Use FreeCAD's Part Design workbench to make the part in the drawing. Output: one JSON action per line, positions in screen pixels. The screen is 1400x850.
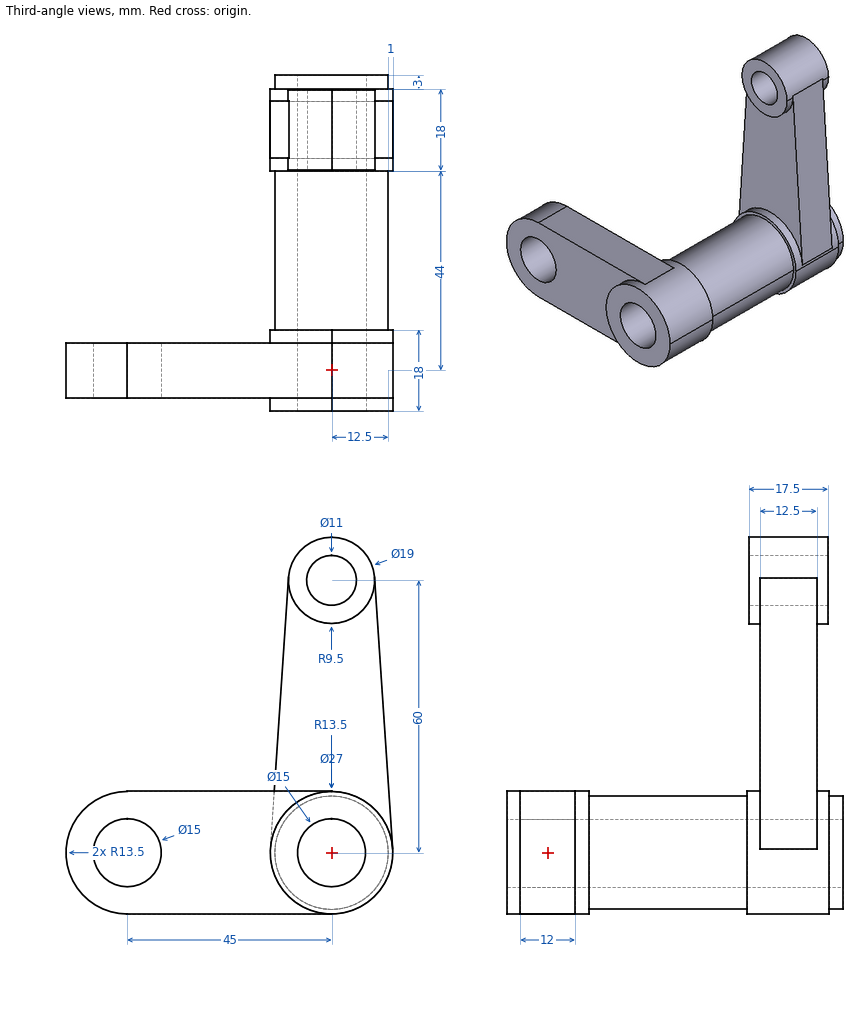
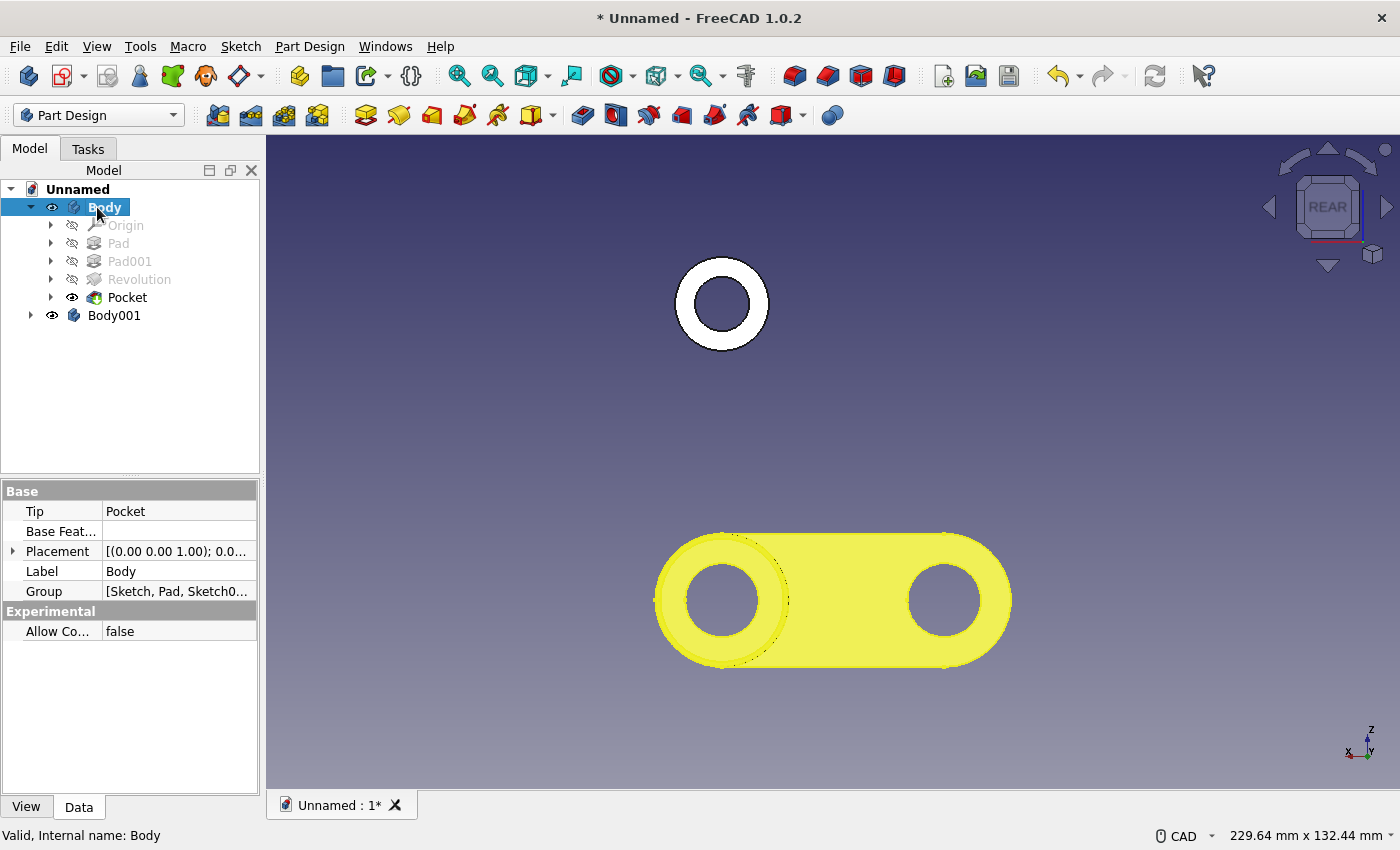
{"action": "left_click", "coordinate": [148, 631]}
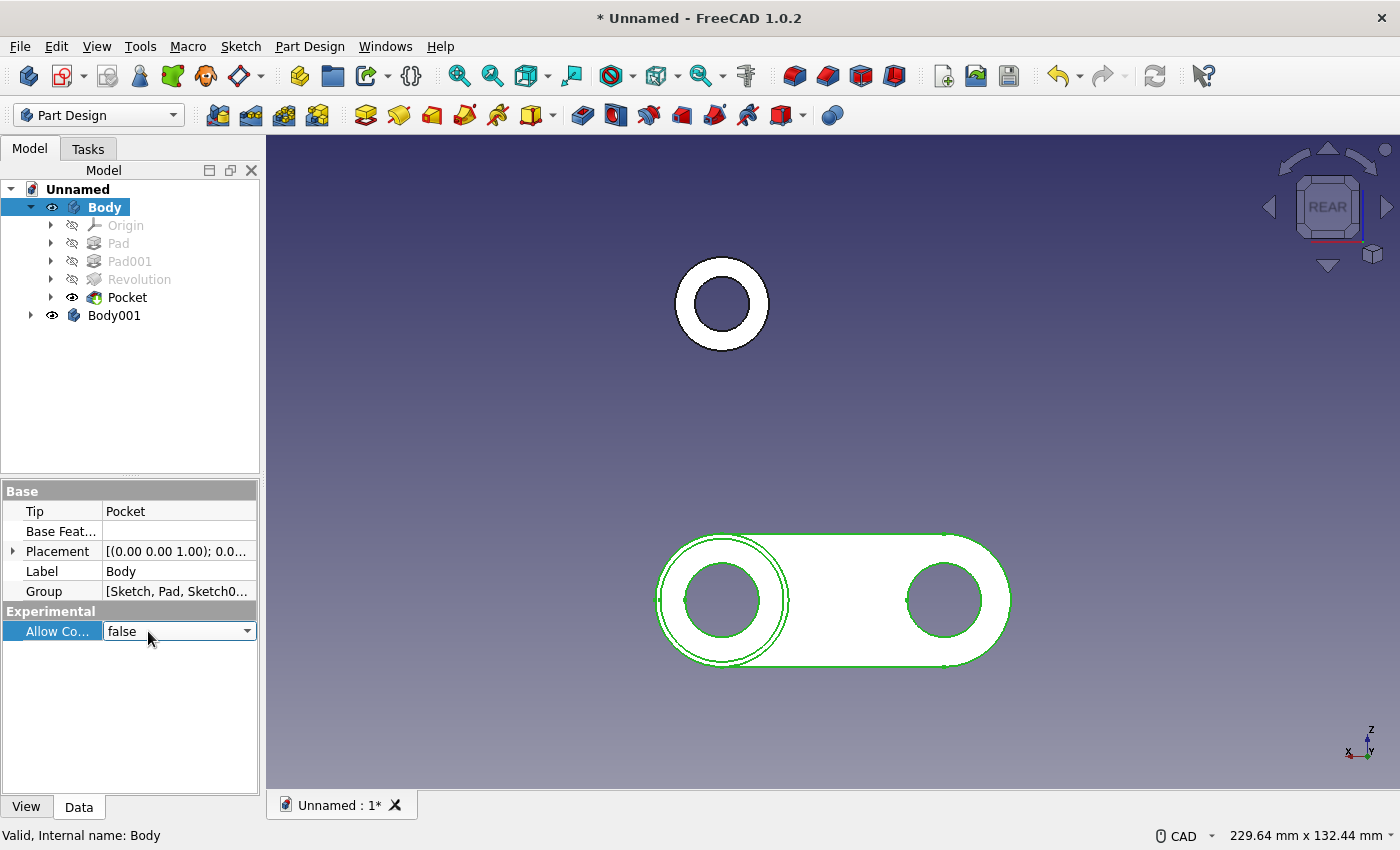
{"action": "left_click", "coordinate": [148, 631]}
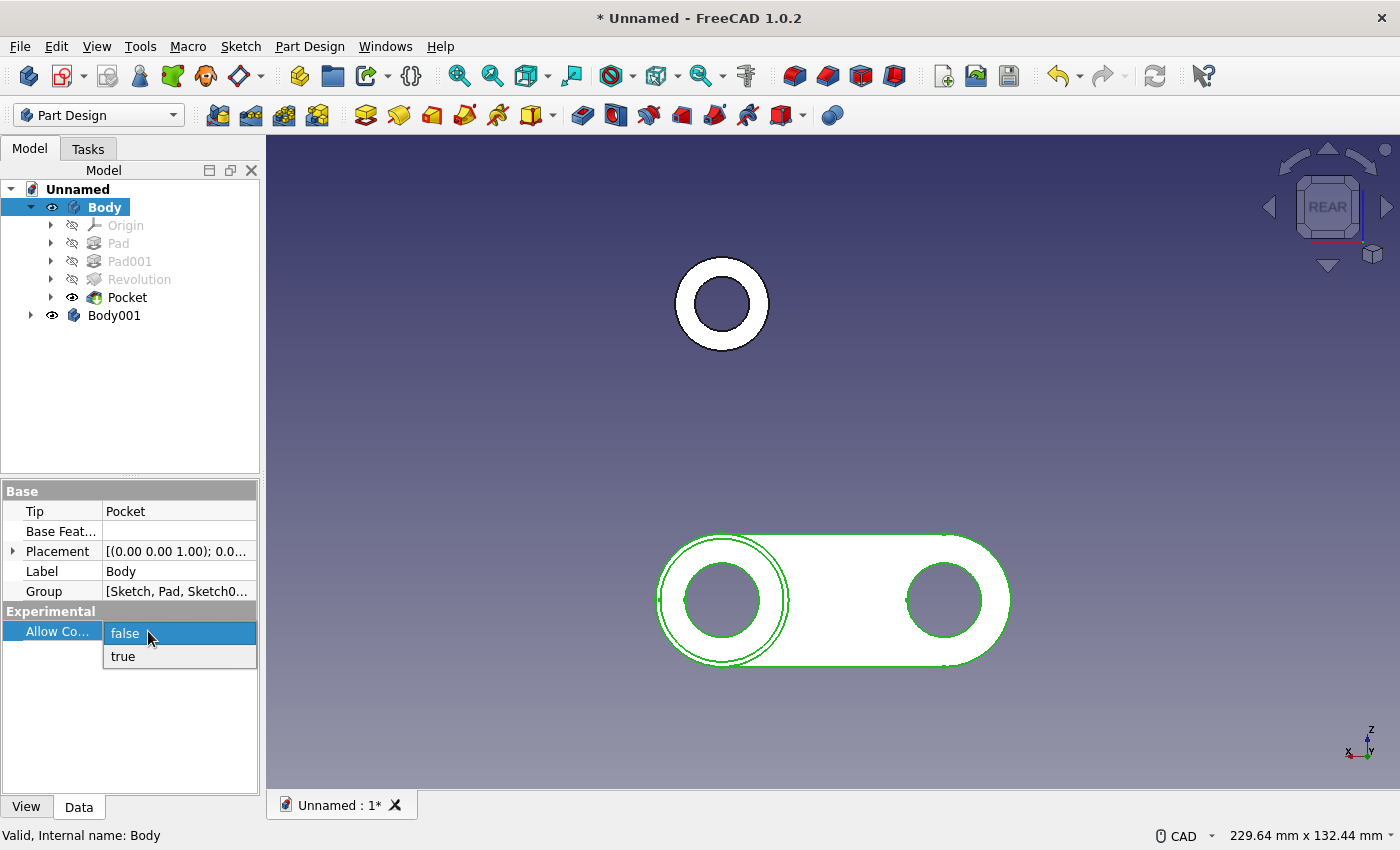
{"action": "left_click", "coordinate": [178, 656]}
{"action": "key", "text": "Return"}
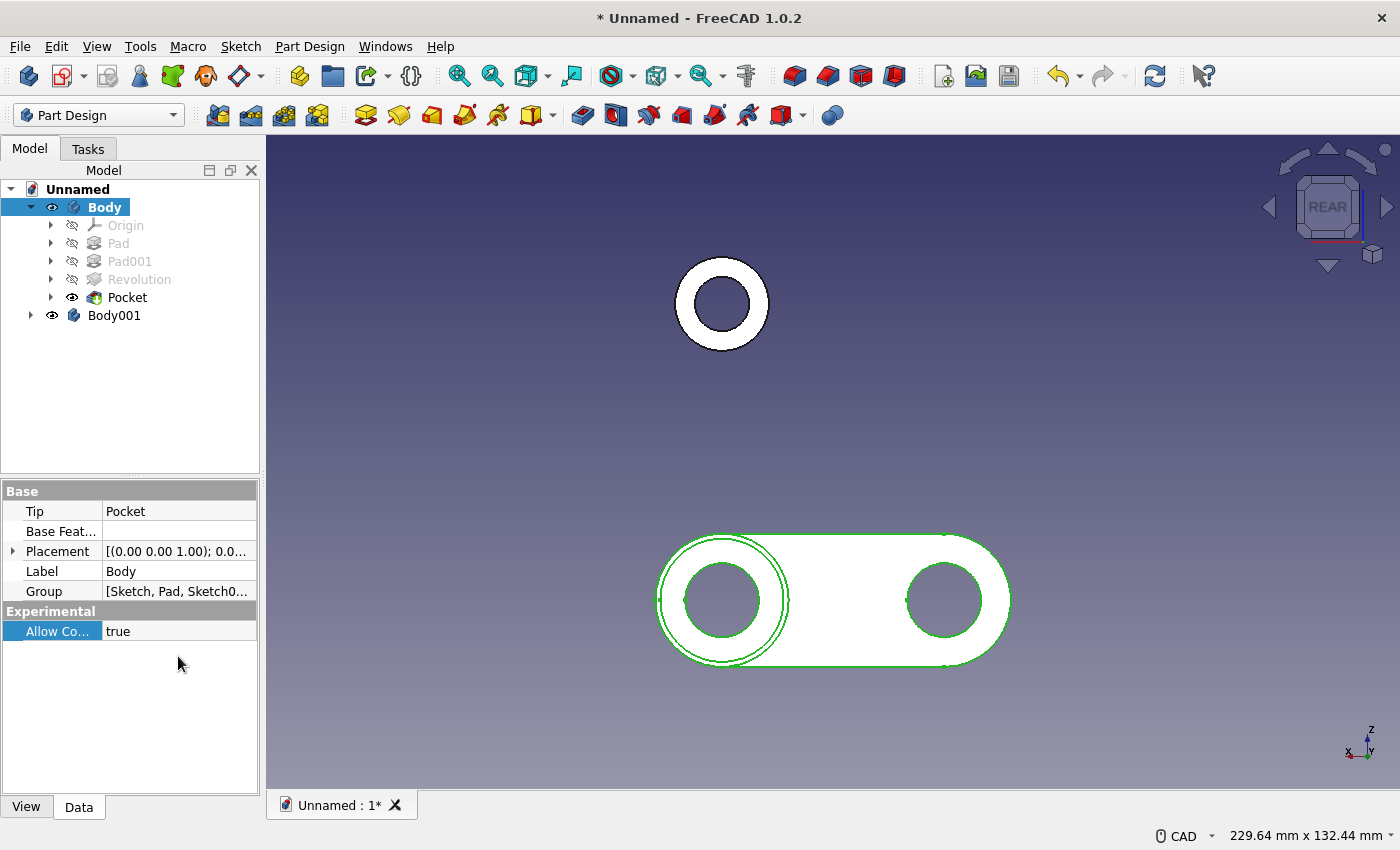
{"action": "left_click", "coordinate": [97, 315]}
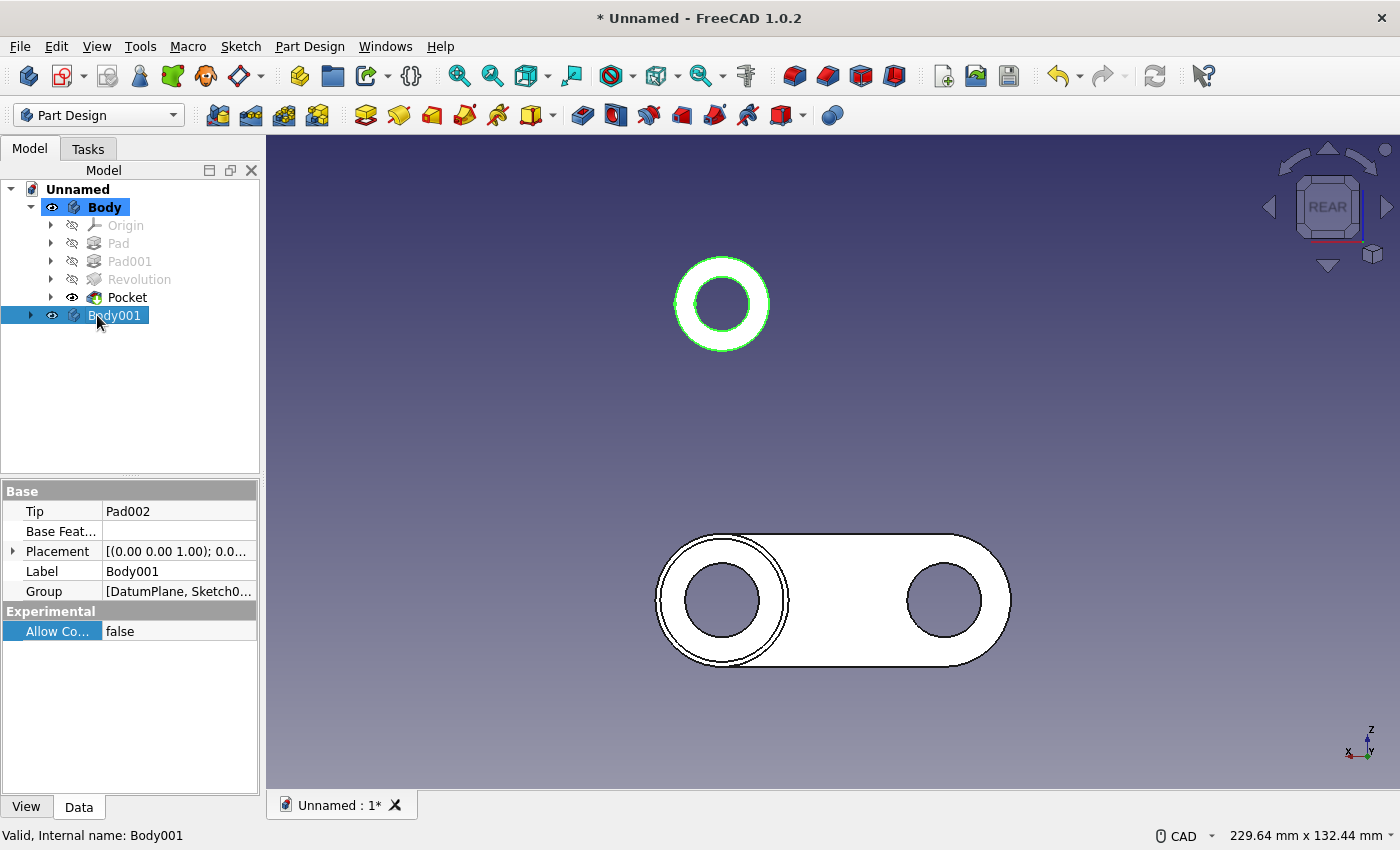
{"action": "left_click", "coordinate": [833, 116]}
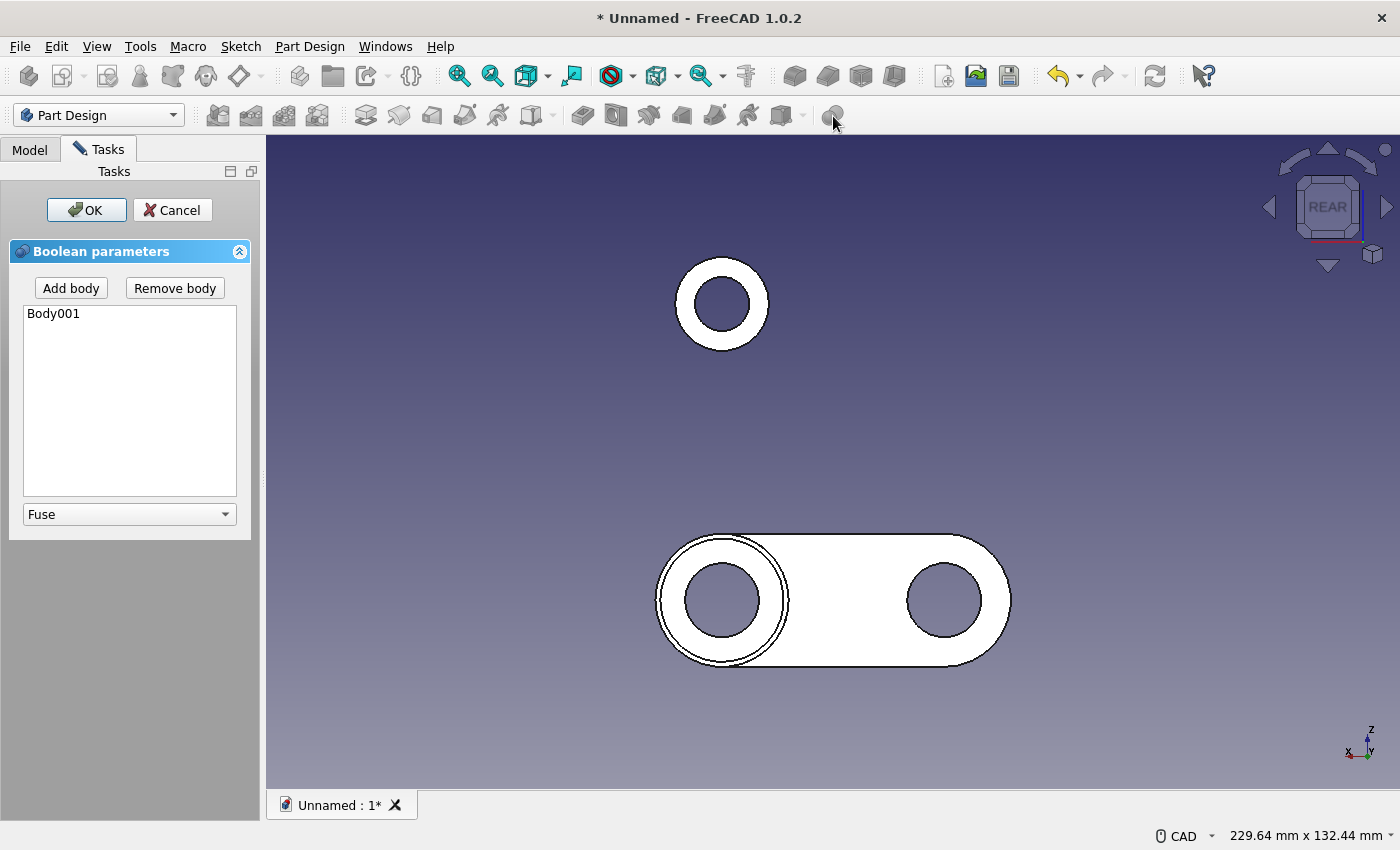
{"action": "left_click", "coordinate": [87, 210]}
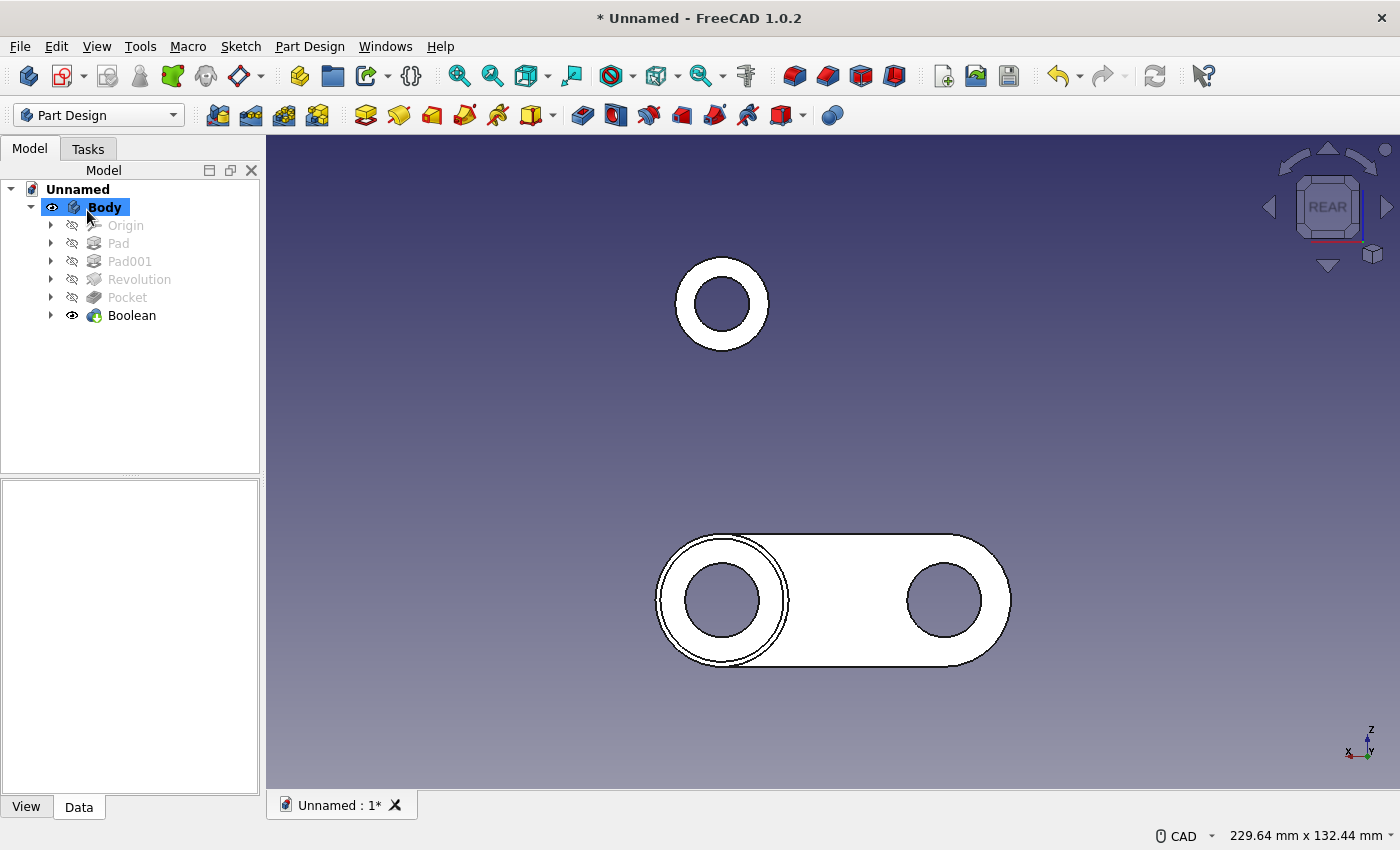
{"action": "left_click", "coordinate": [51, 225]}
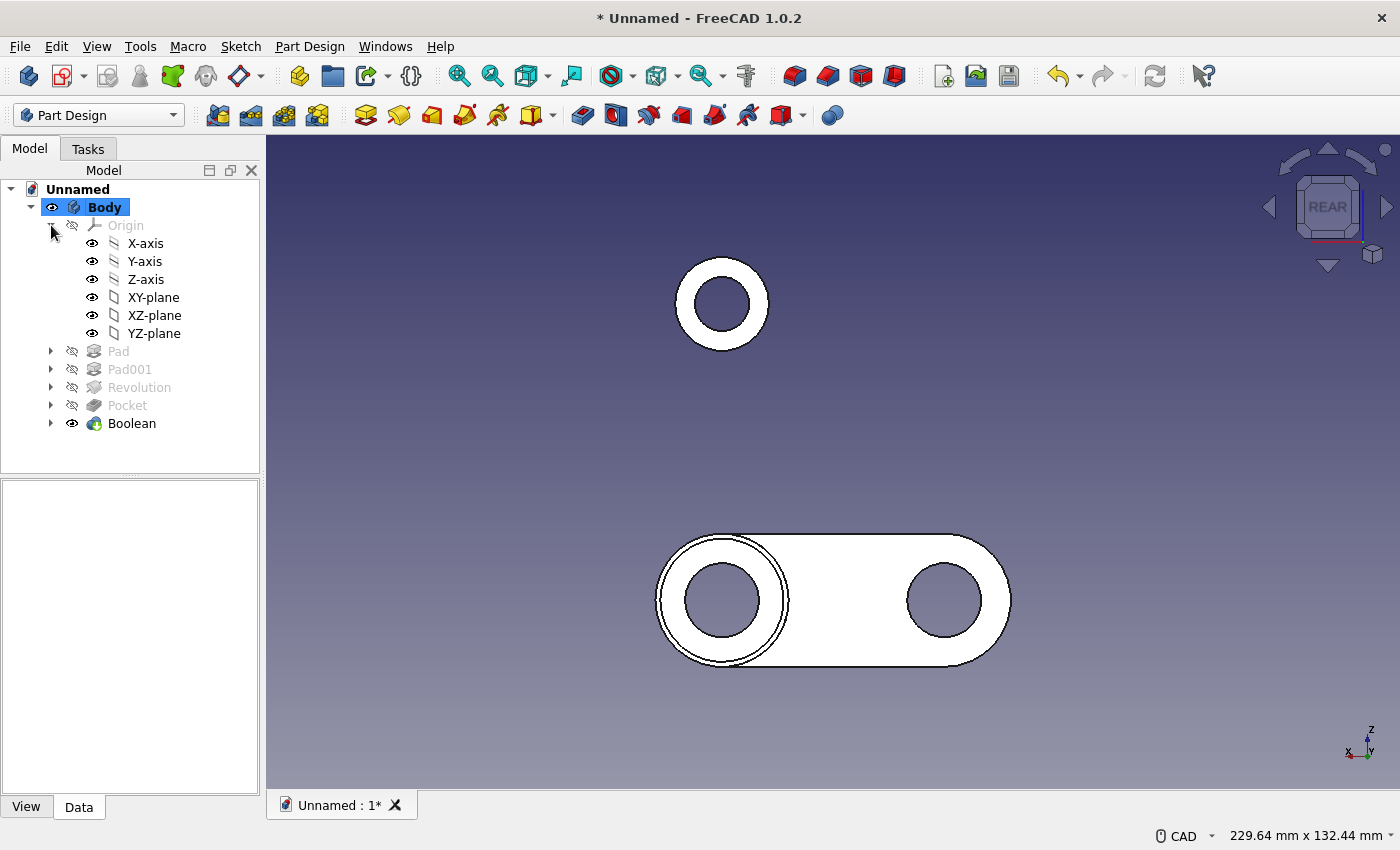
{"action": "left_click", "coordinate": [137, 315]}